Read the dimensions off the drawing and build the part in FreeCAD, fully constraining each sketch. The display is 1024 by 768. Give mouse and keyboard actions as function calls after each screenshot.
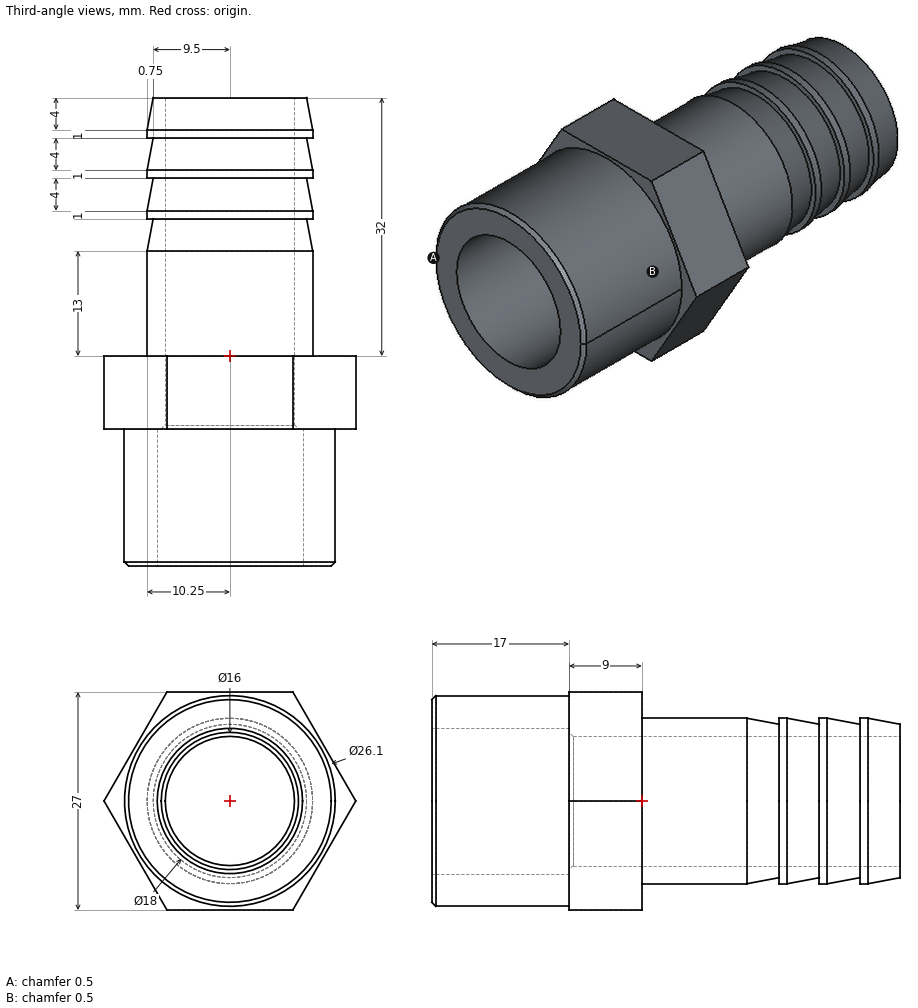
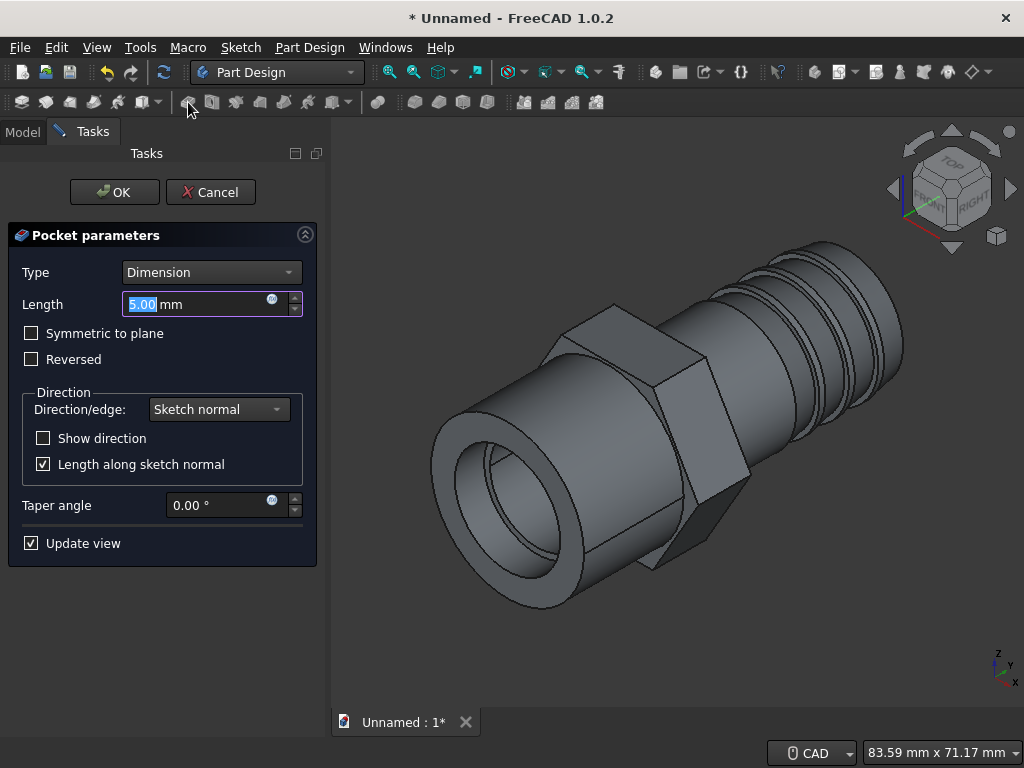
text(17)
key(Tab)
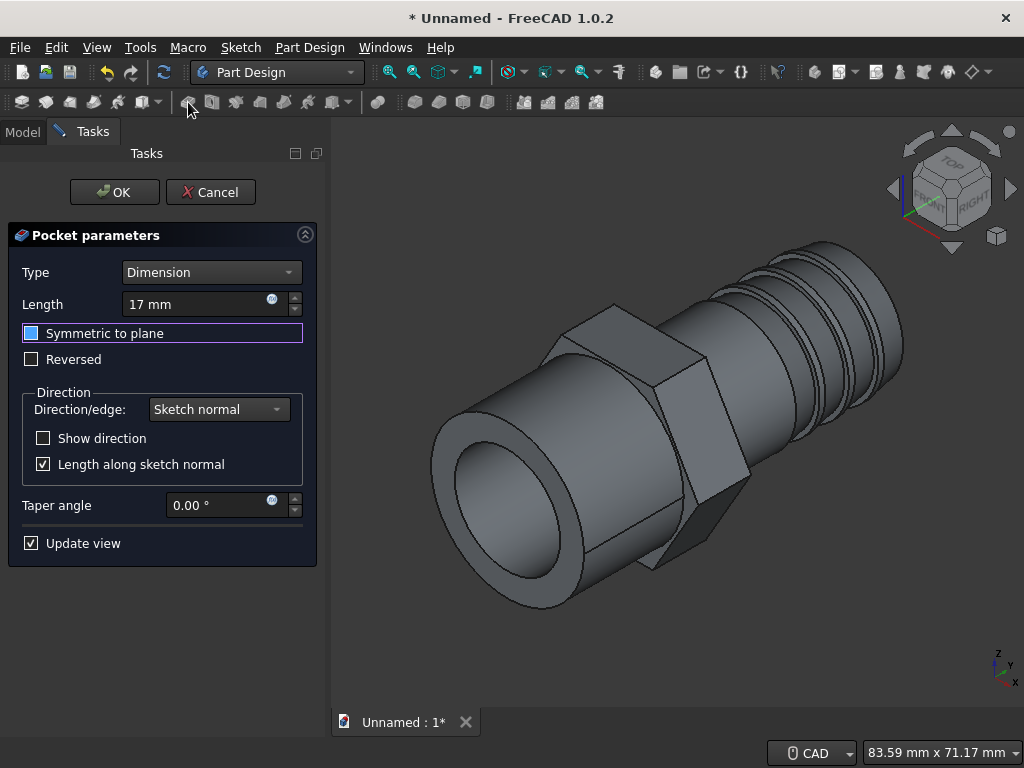
click(115, 192)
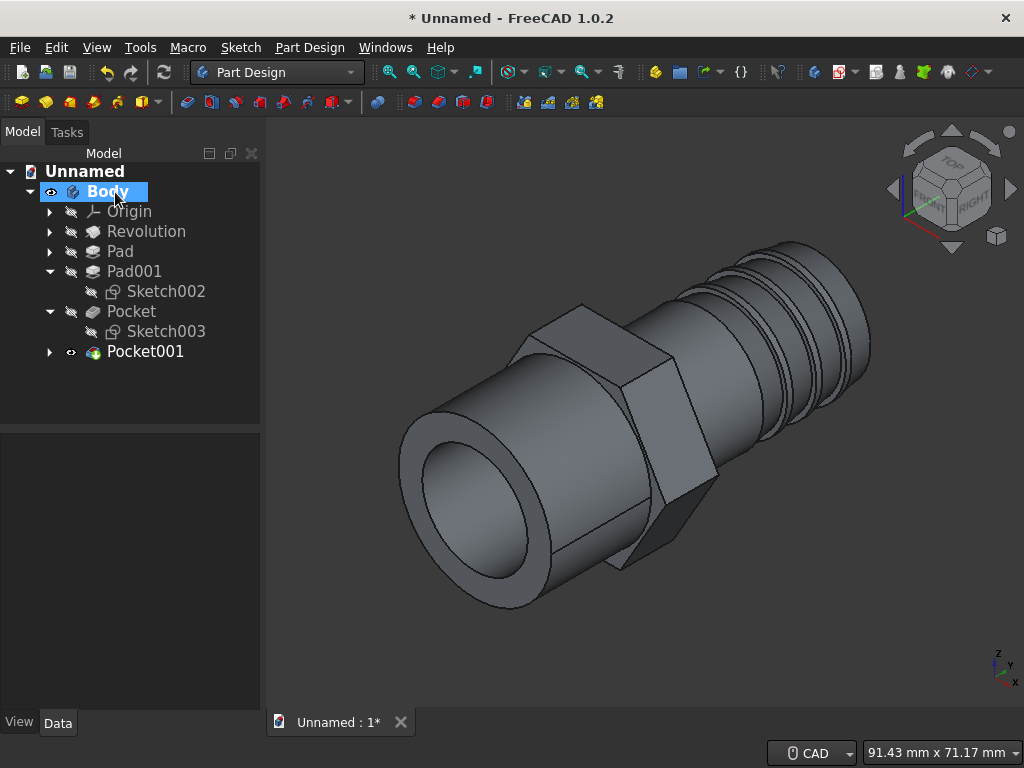
click(451, 411)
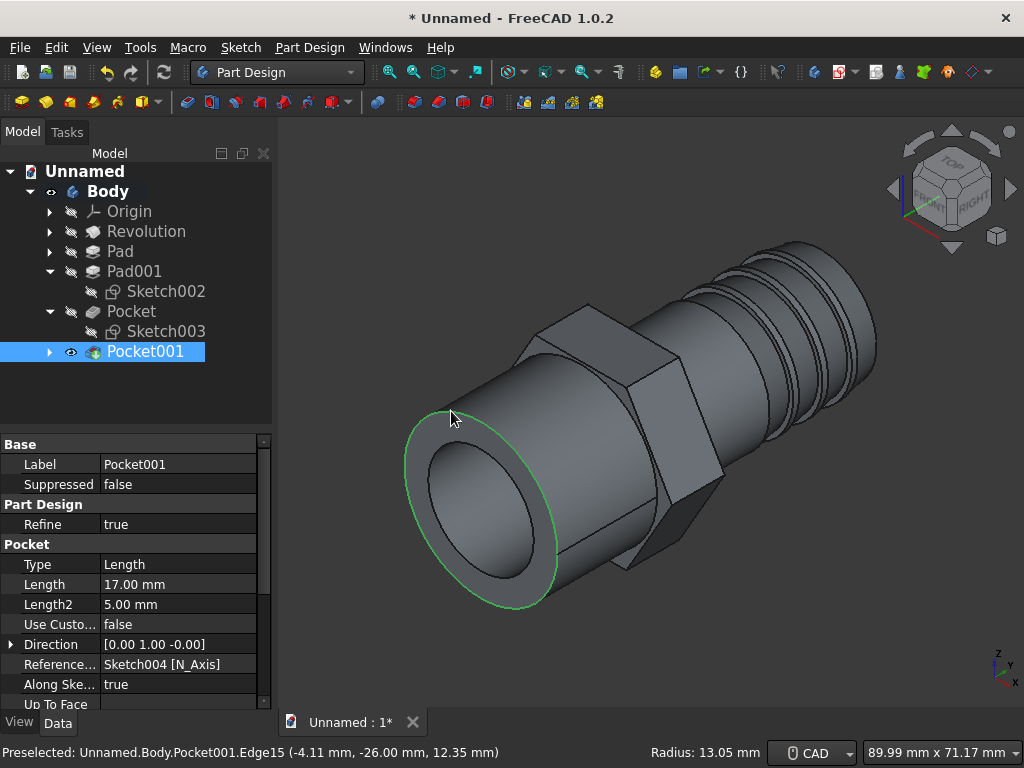
click(440, 102)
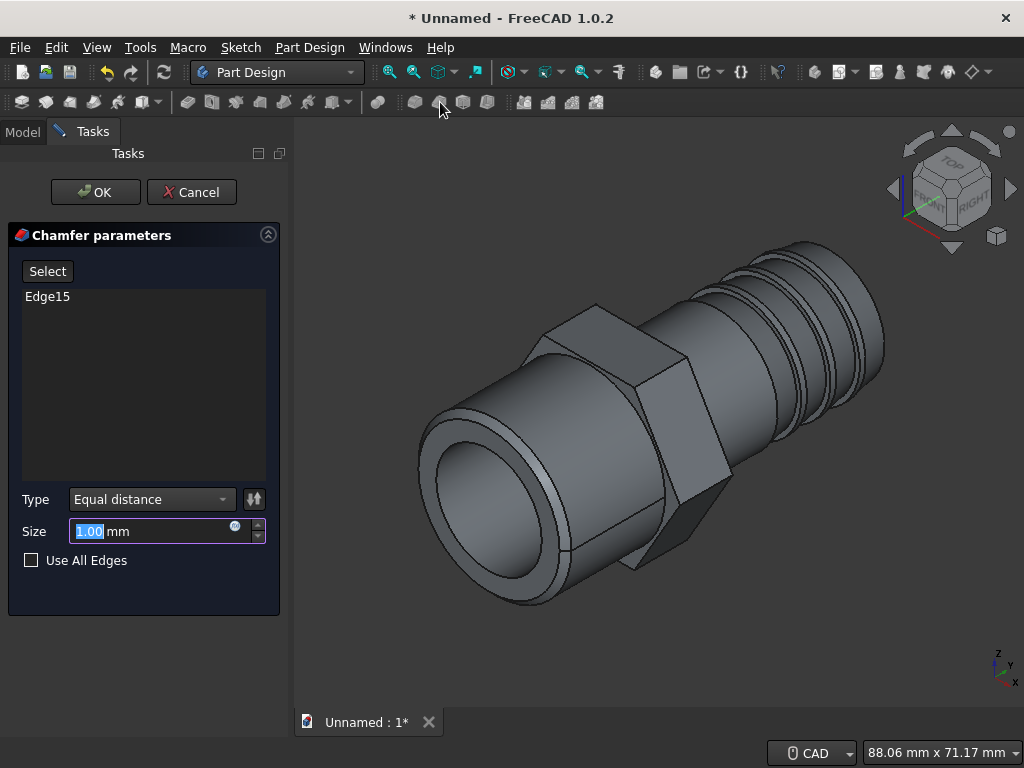
text(0.5)
key(Tab)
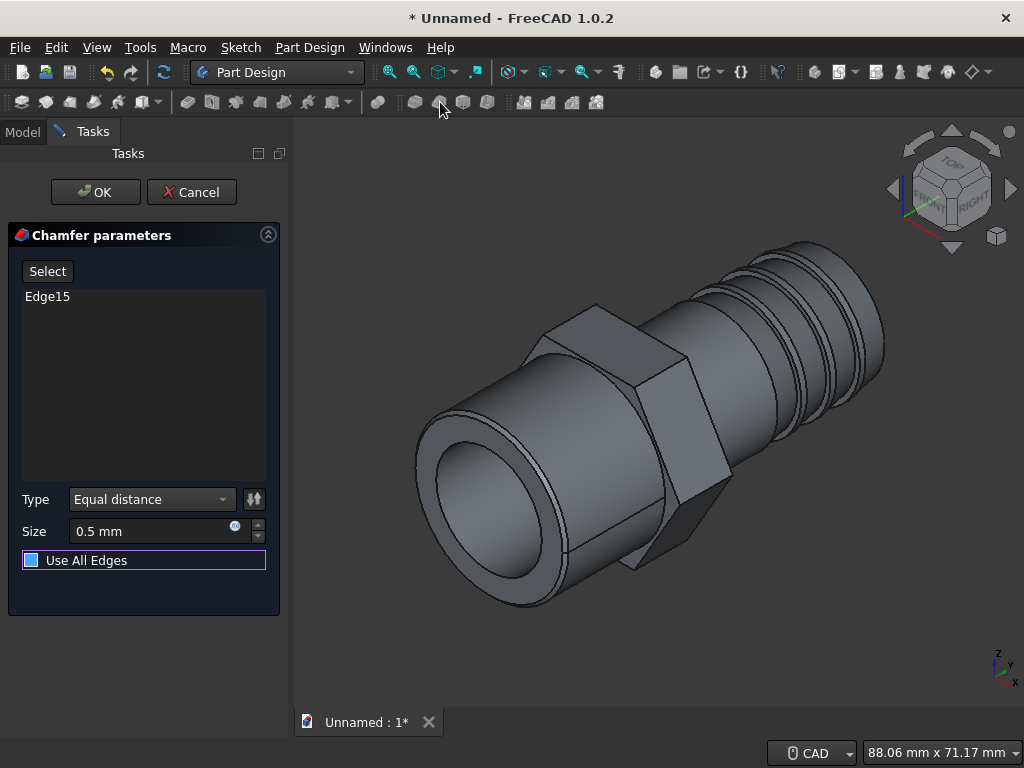
click(96, 192)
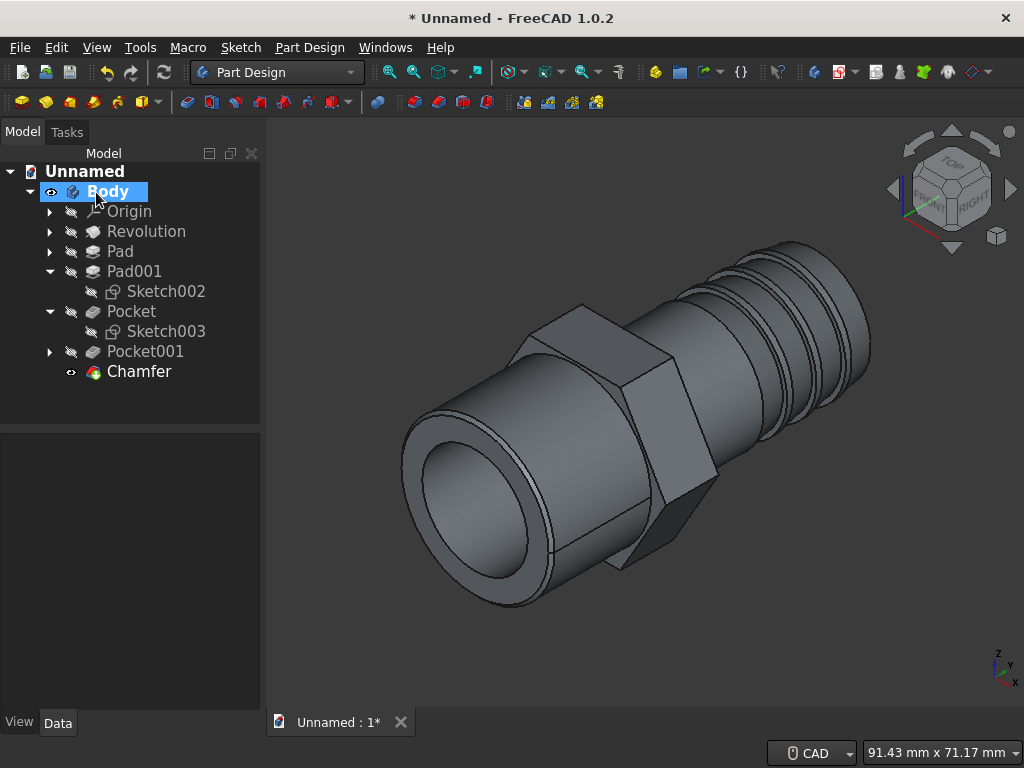
key(2)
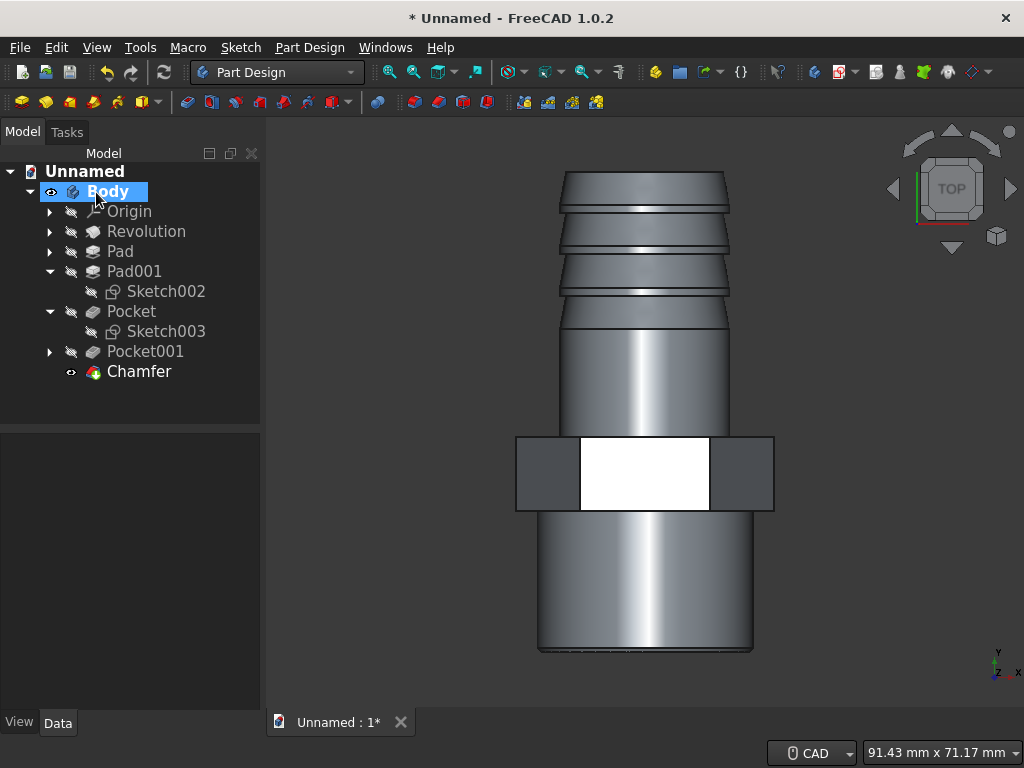
key(0)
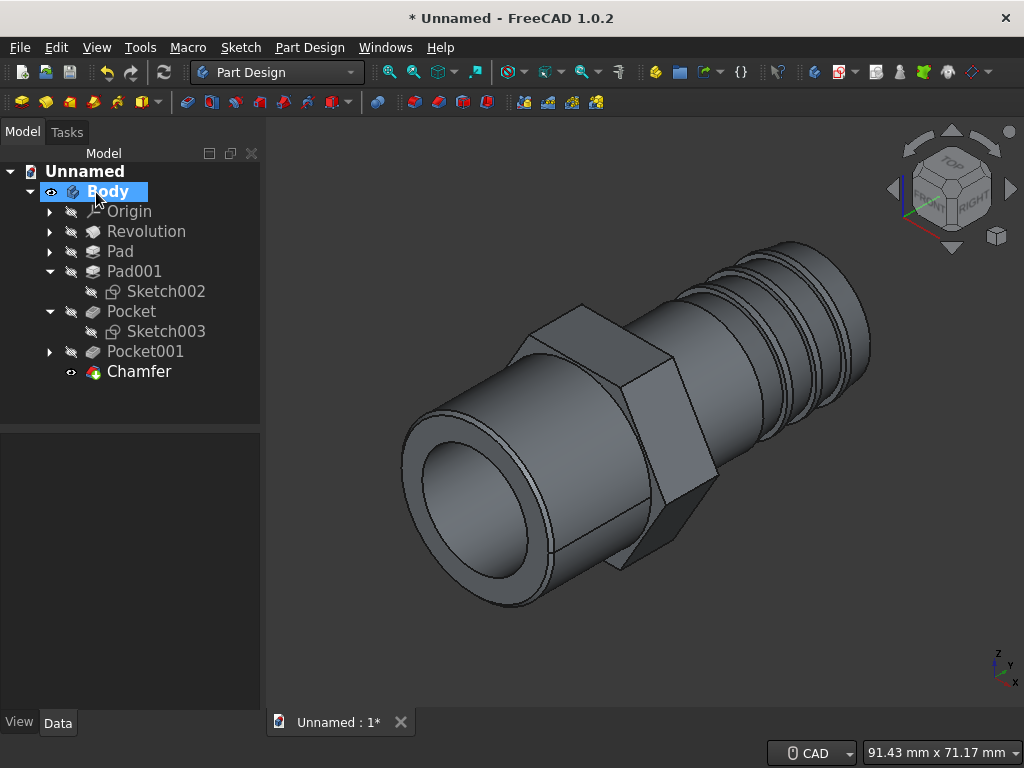
key(1)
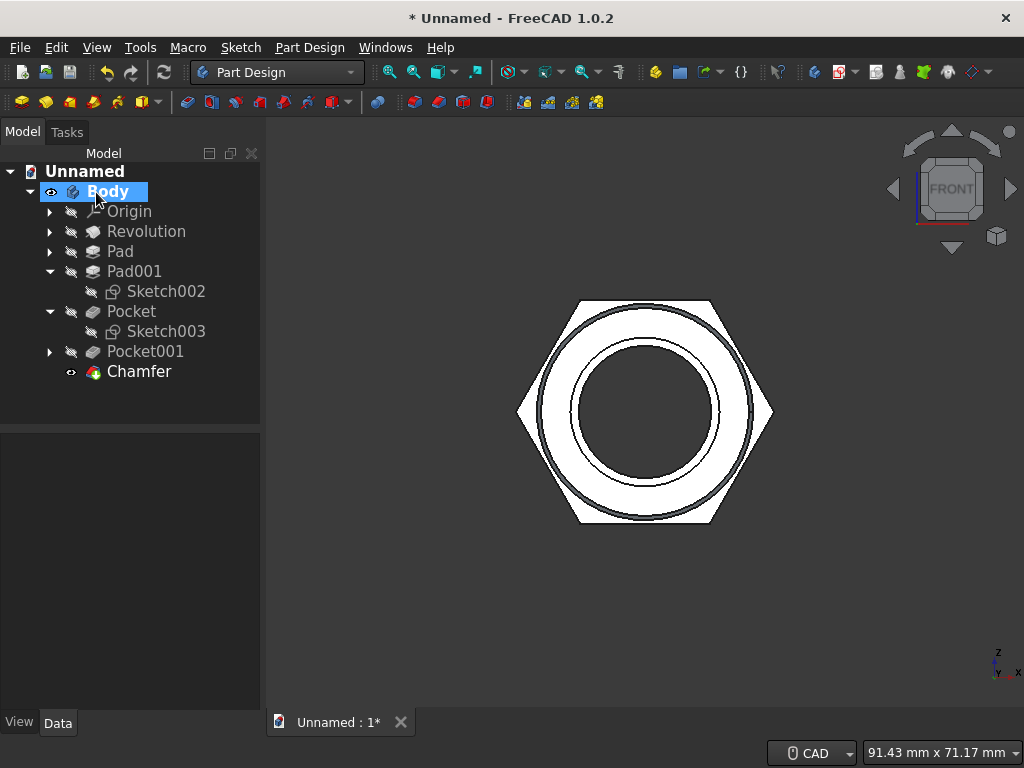
key(v)
key(f)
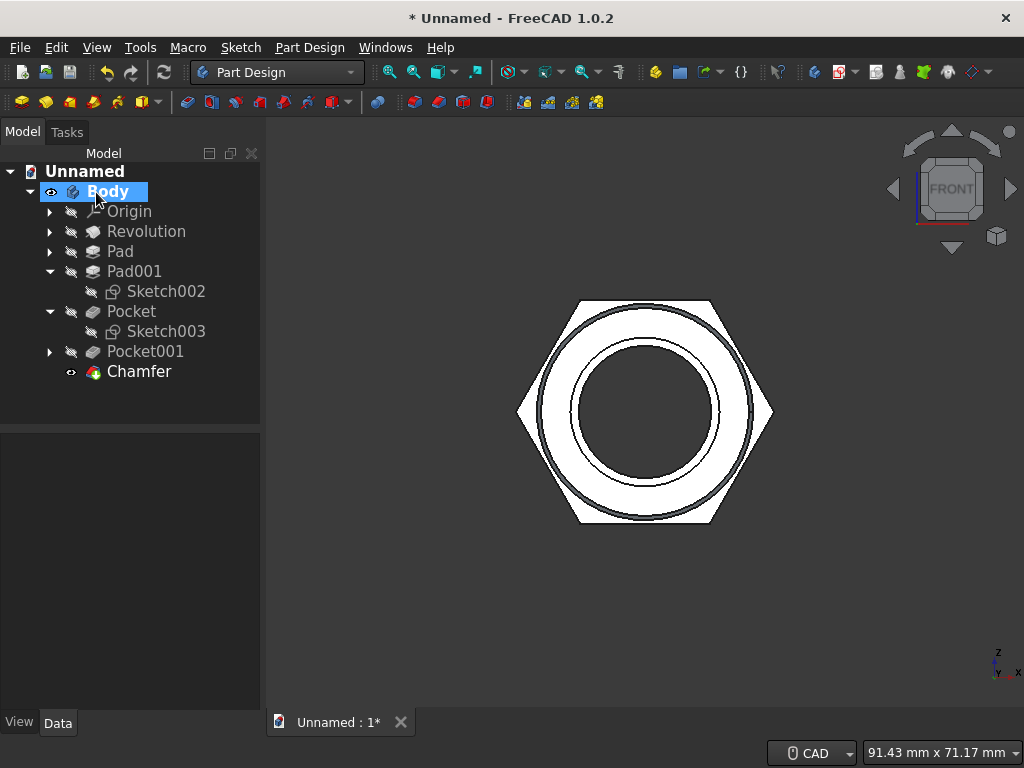
click(711, 411)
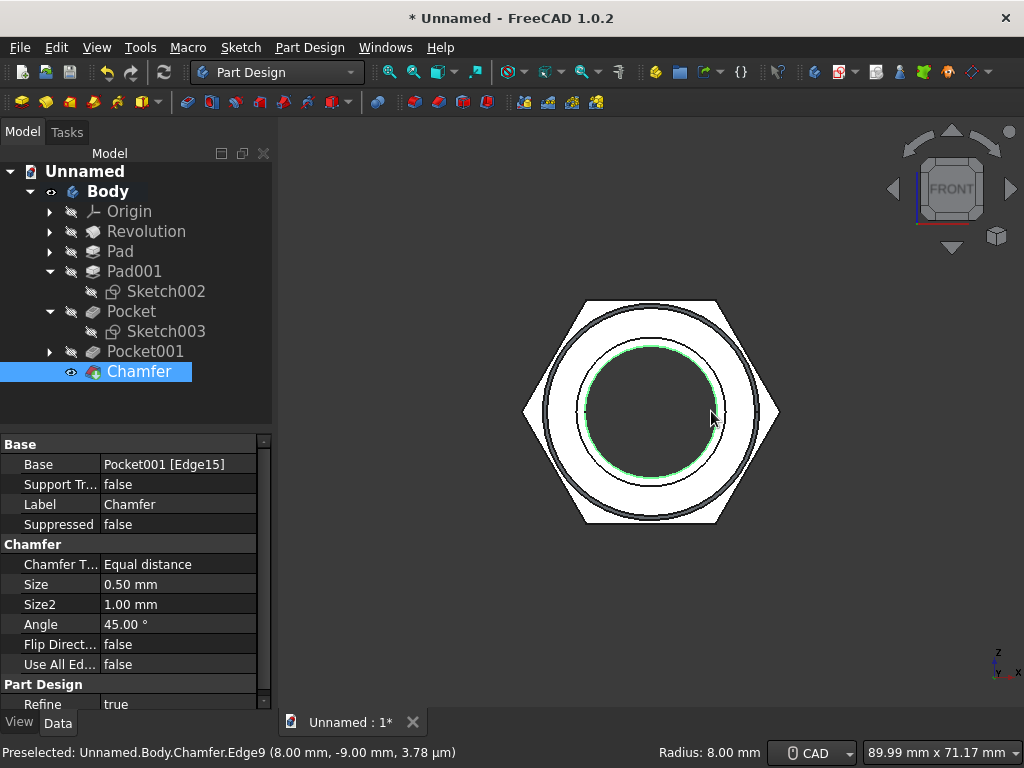
click(440, 102)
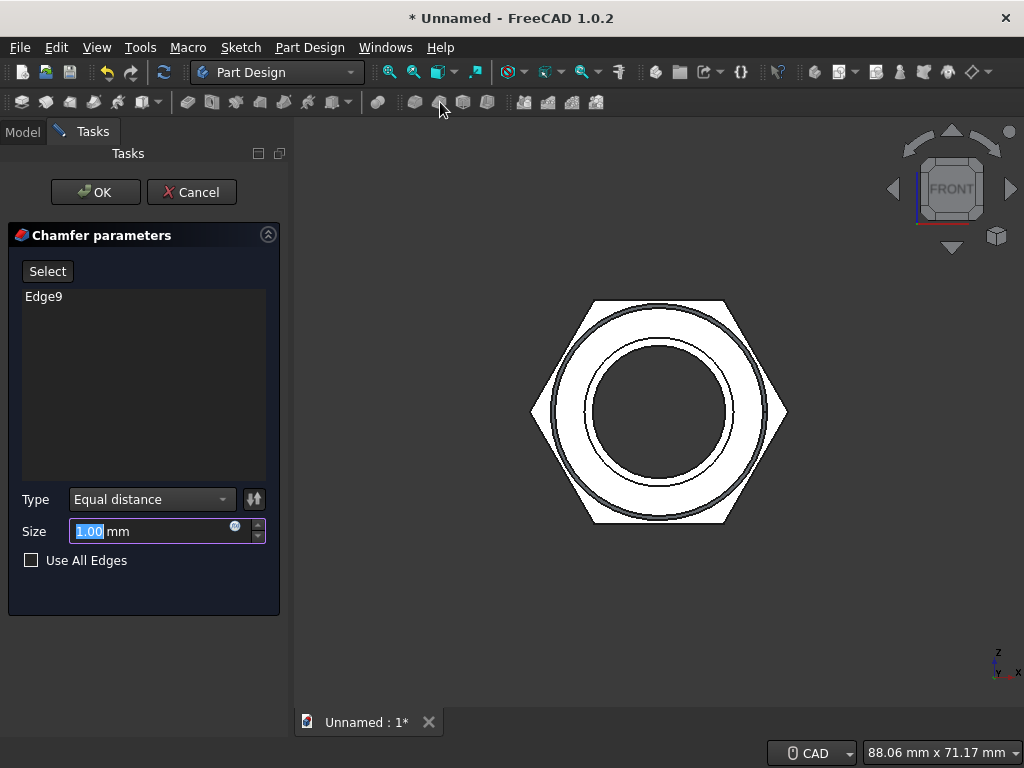
text(0.5)
key(Tab)